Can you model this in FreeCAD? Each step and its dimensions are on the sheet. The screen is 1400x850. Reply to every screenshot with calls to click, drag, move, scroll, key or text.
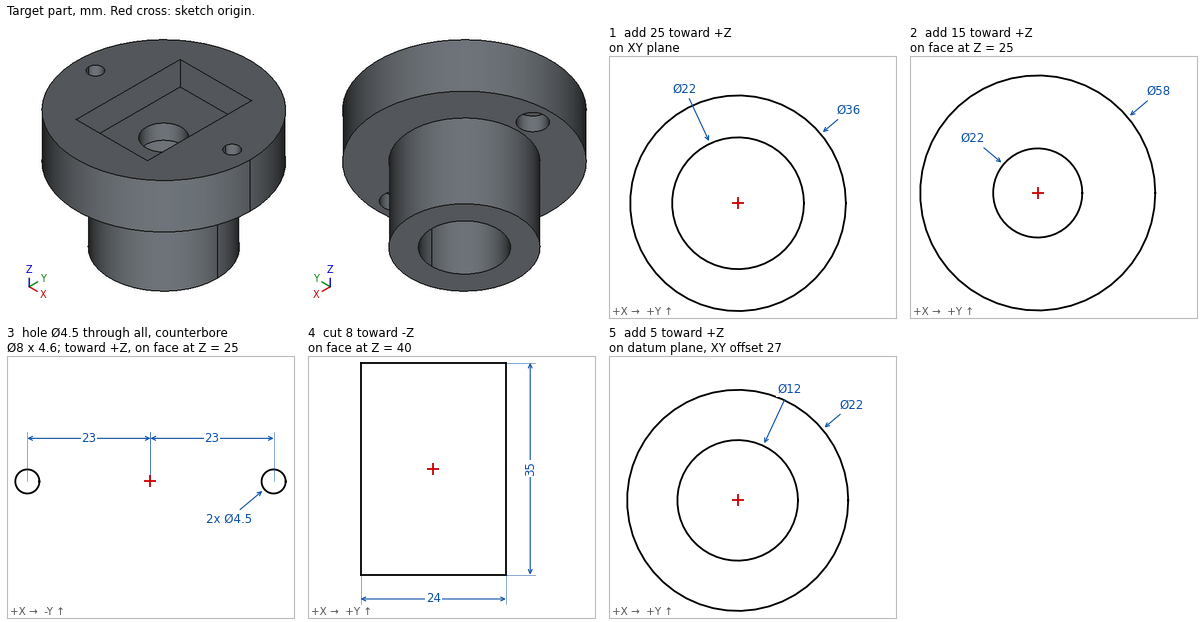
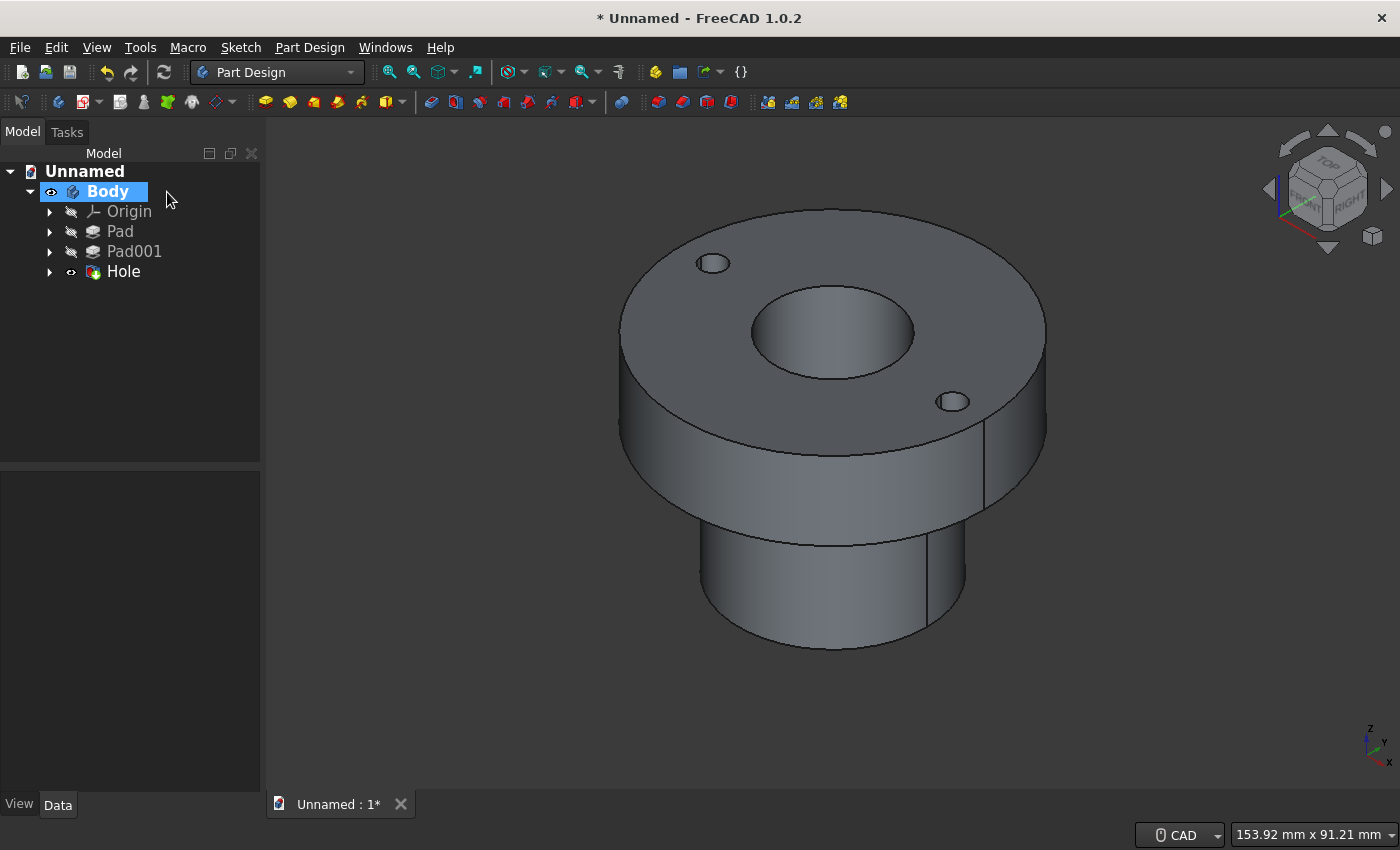
click(962, 357)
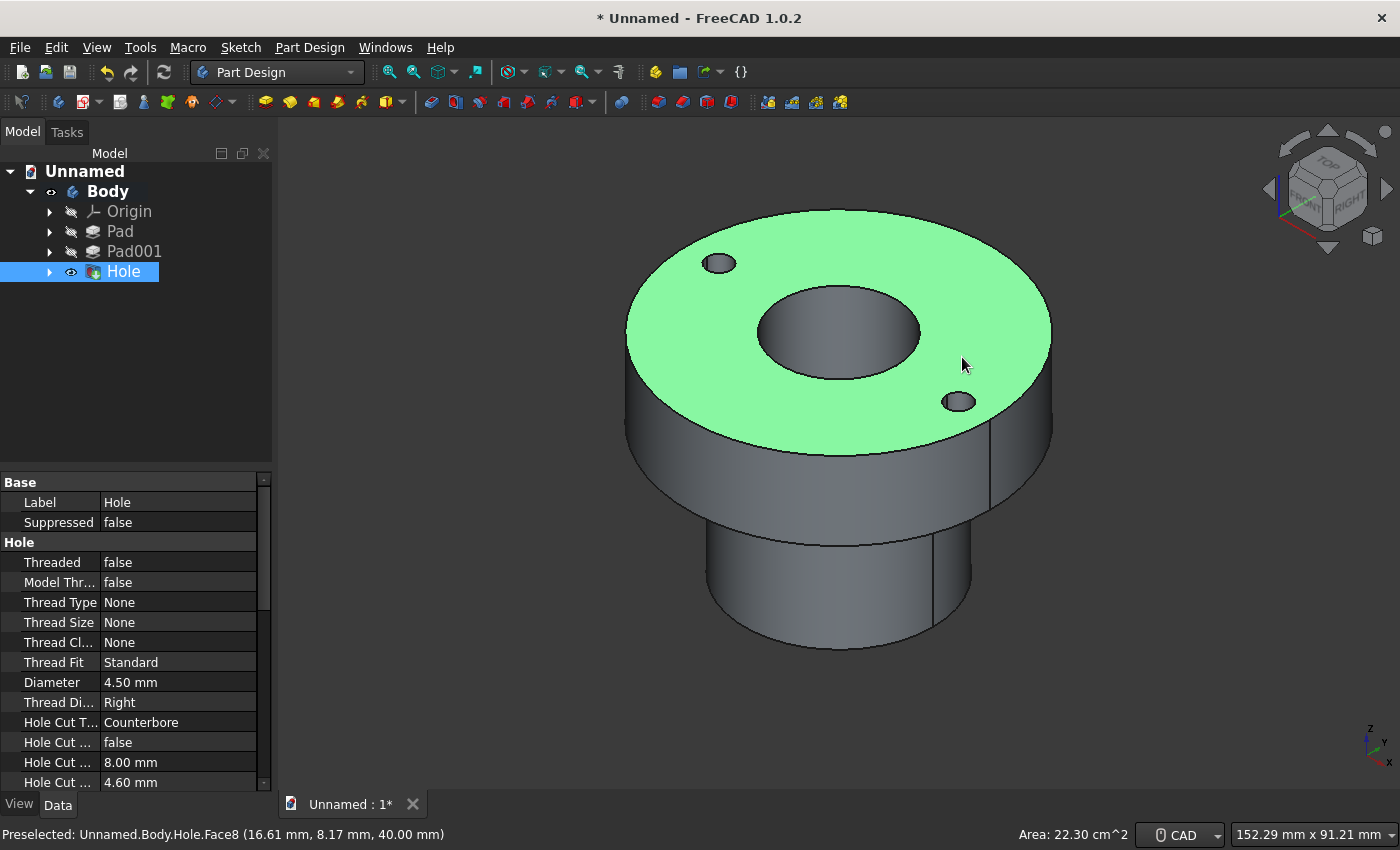
click(84, 102)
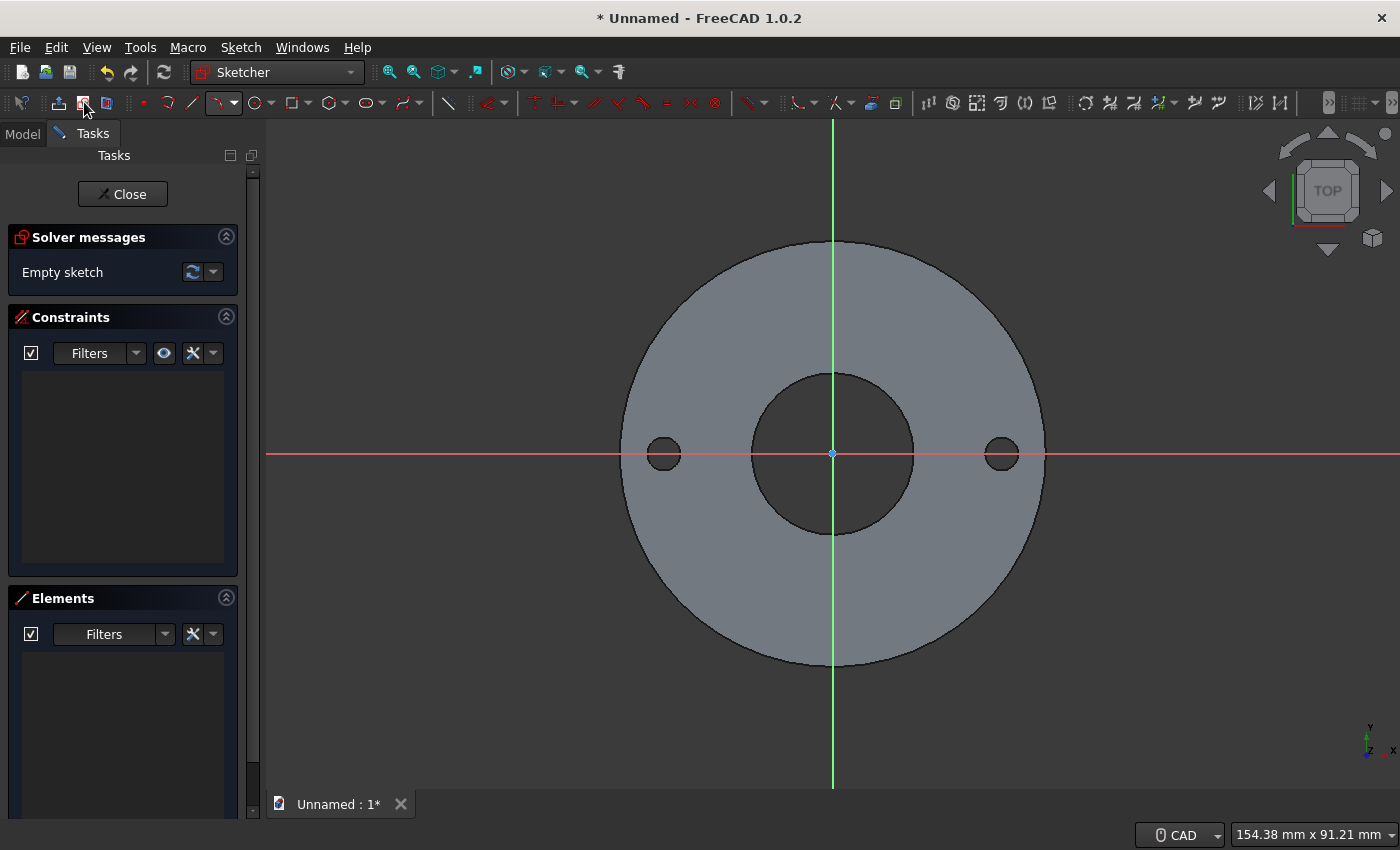
scroll(916, 454, up, 3)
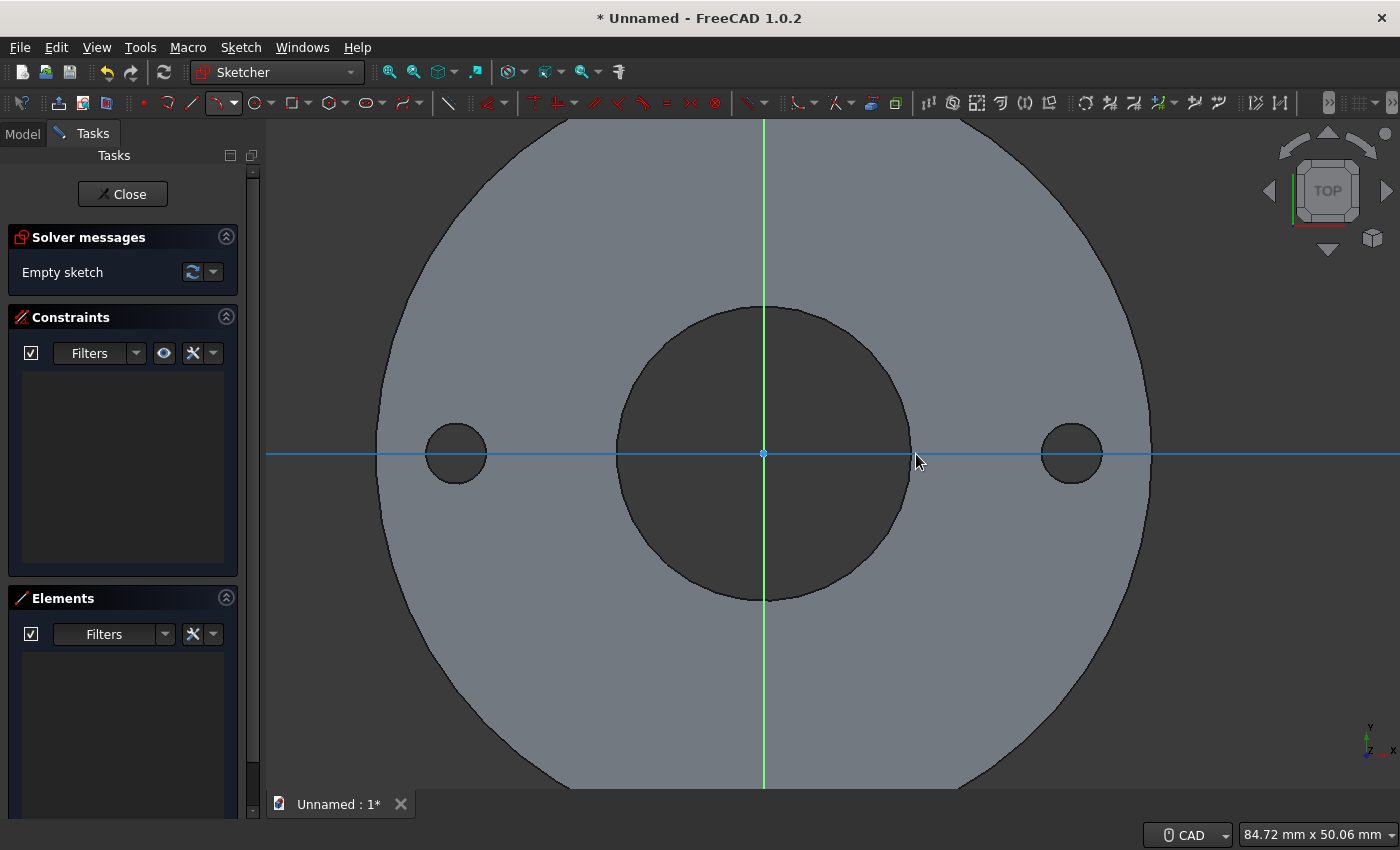
key(g)
key(v)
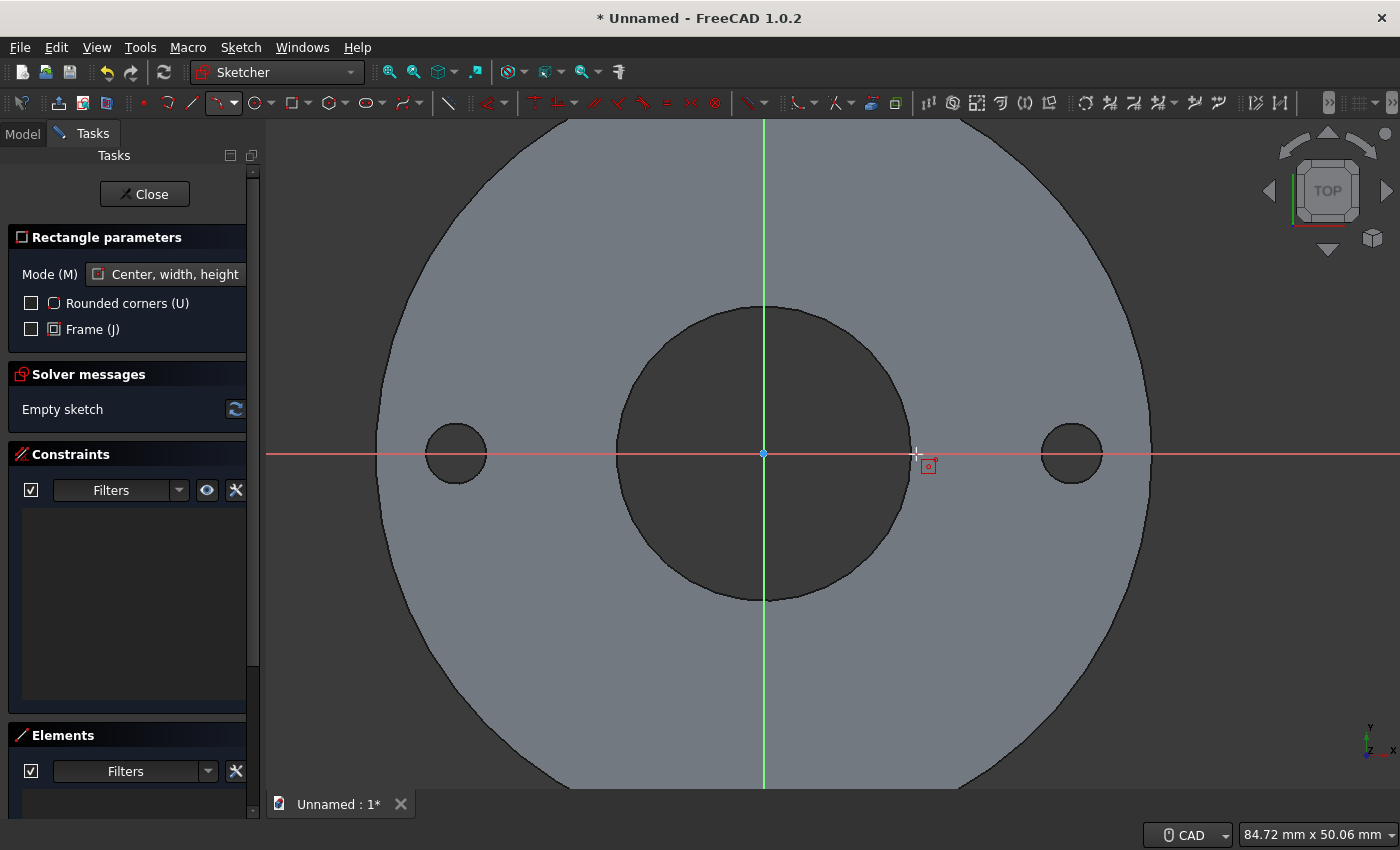
click(764, 454)
click(925, 219)
key(Escape)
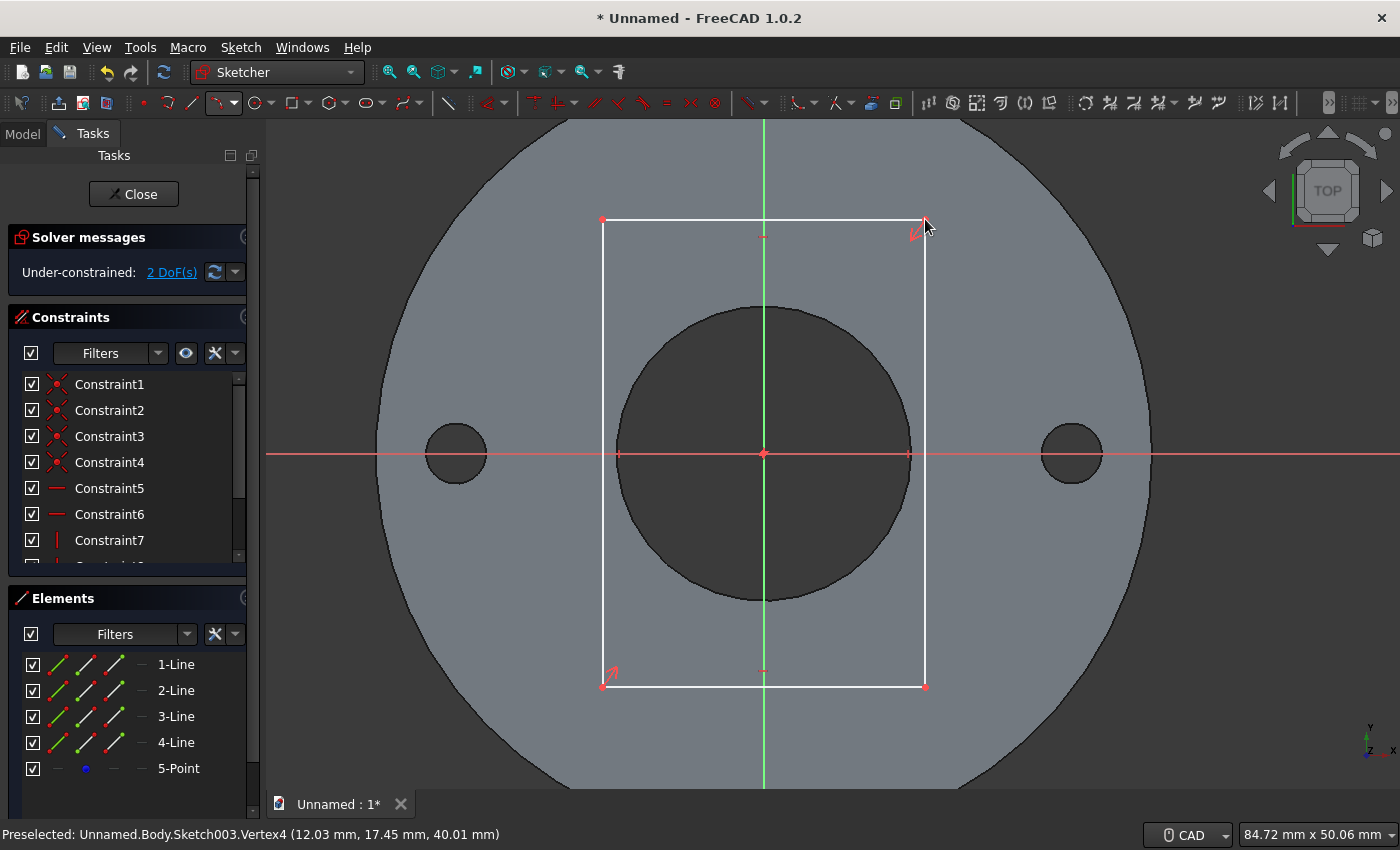
key(d)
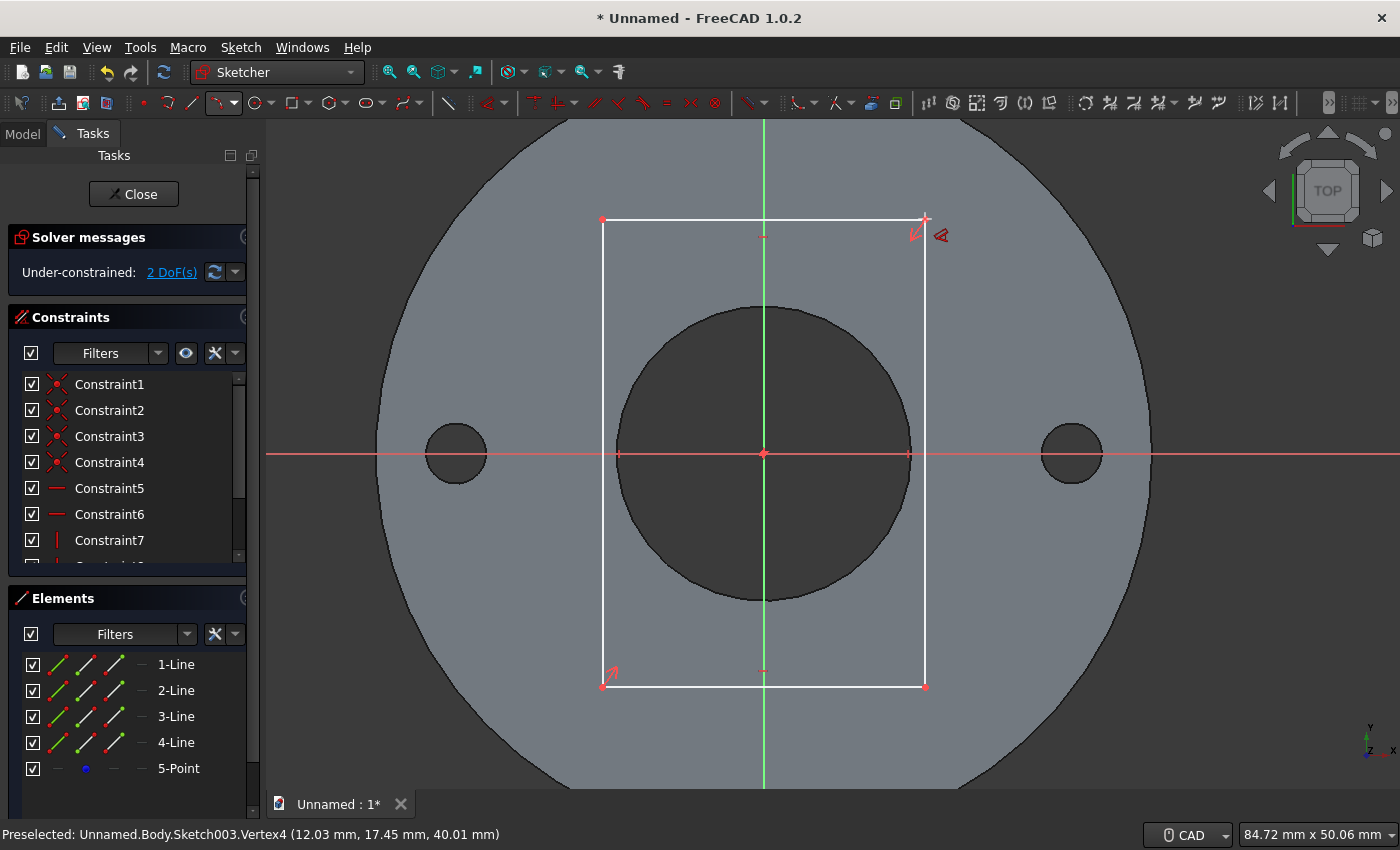
click(700, 687)
click(690, 721)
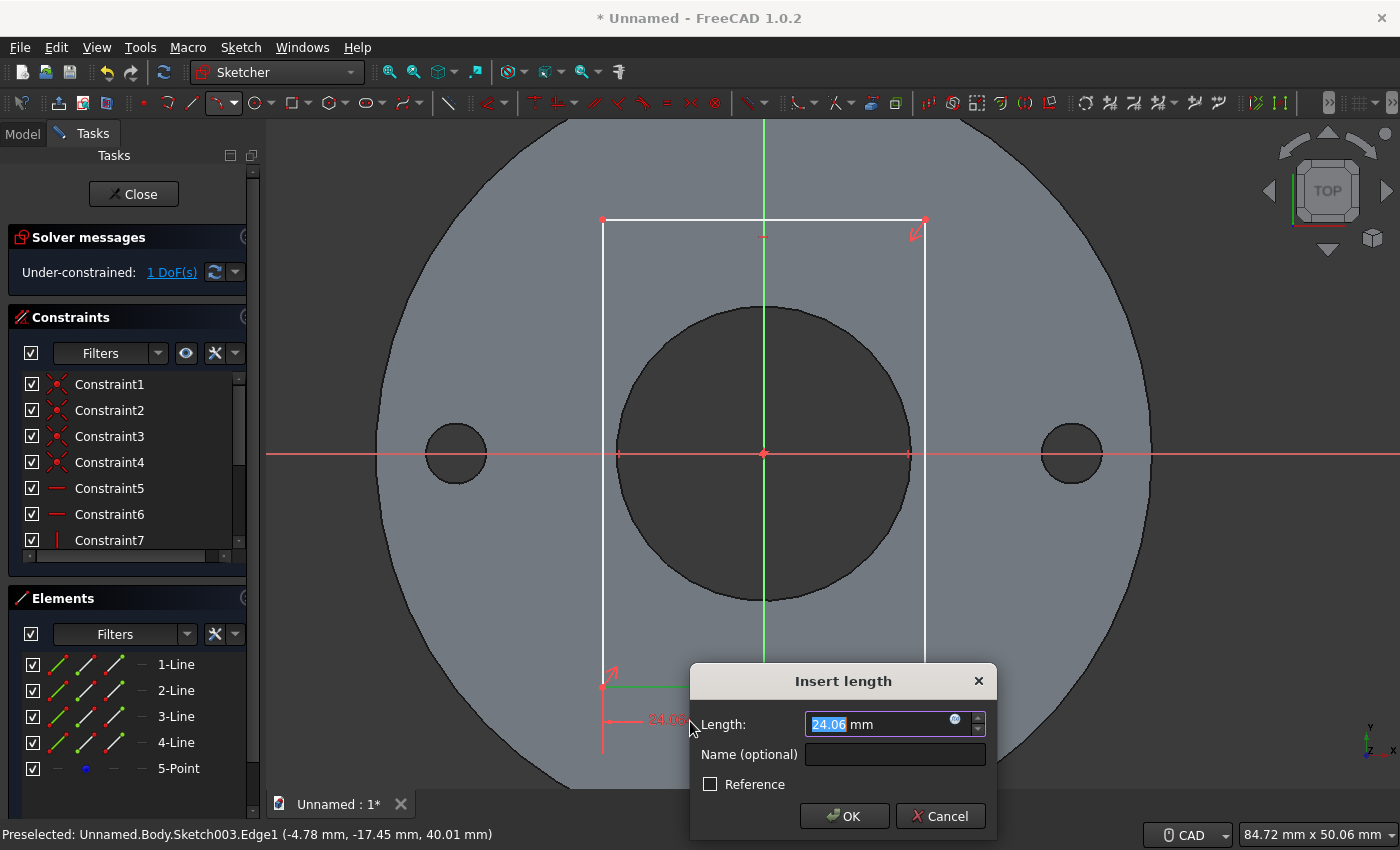
text(24)
key(Return)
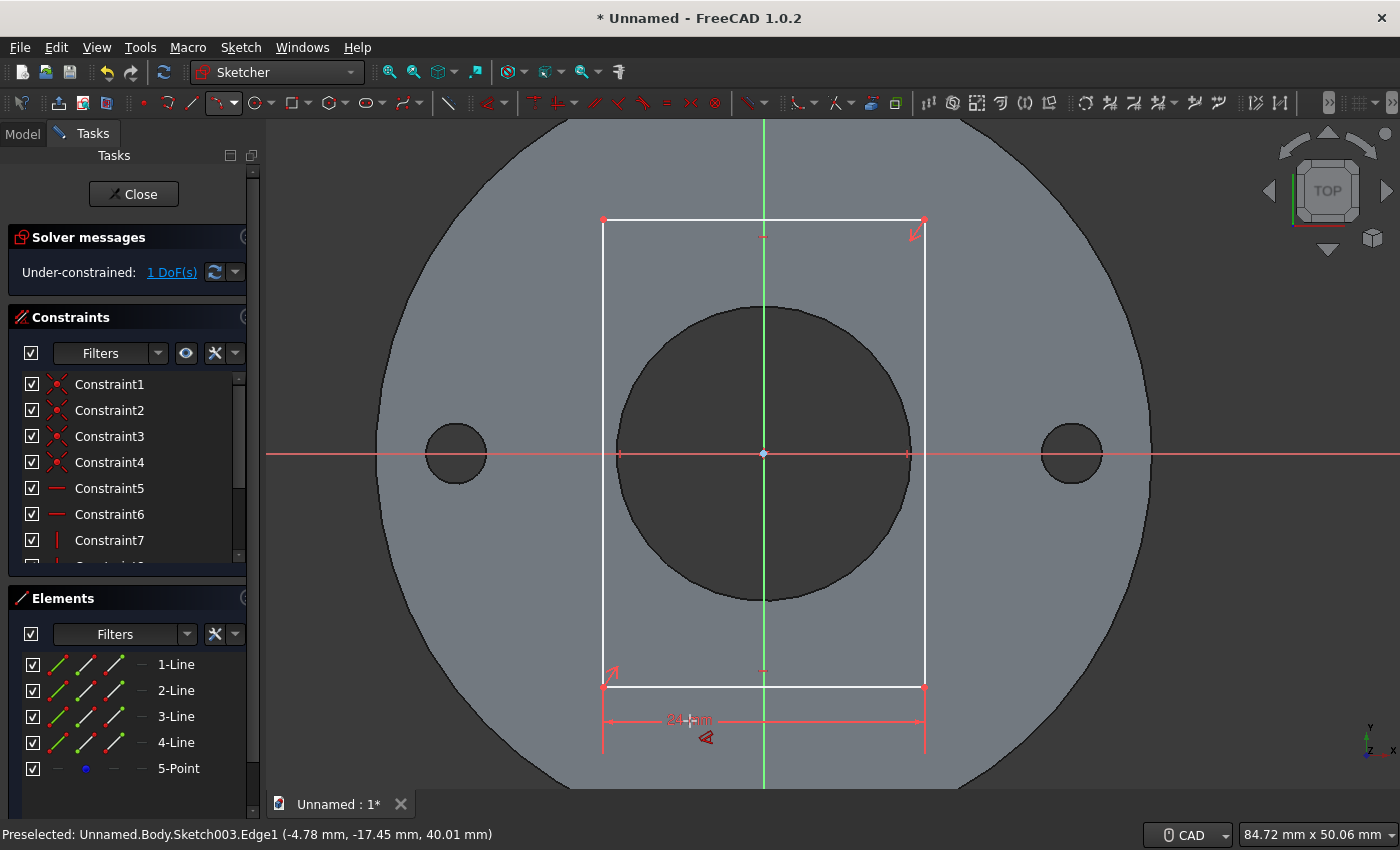
click(925, 547)
click(959, 346)